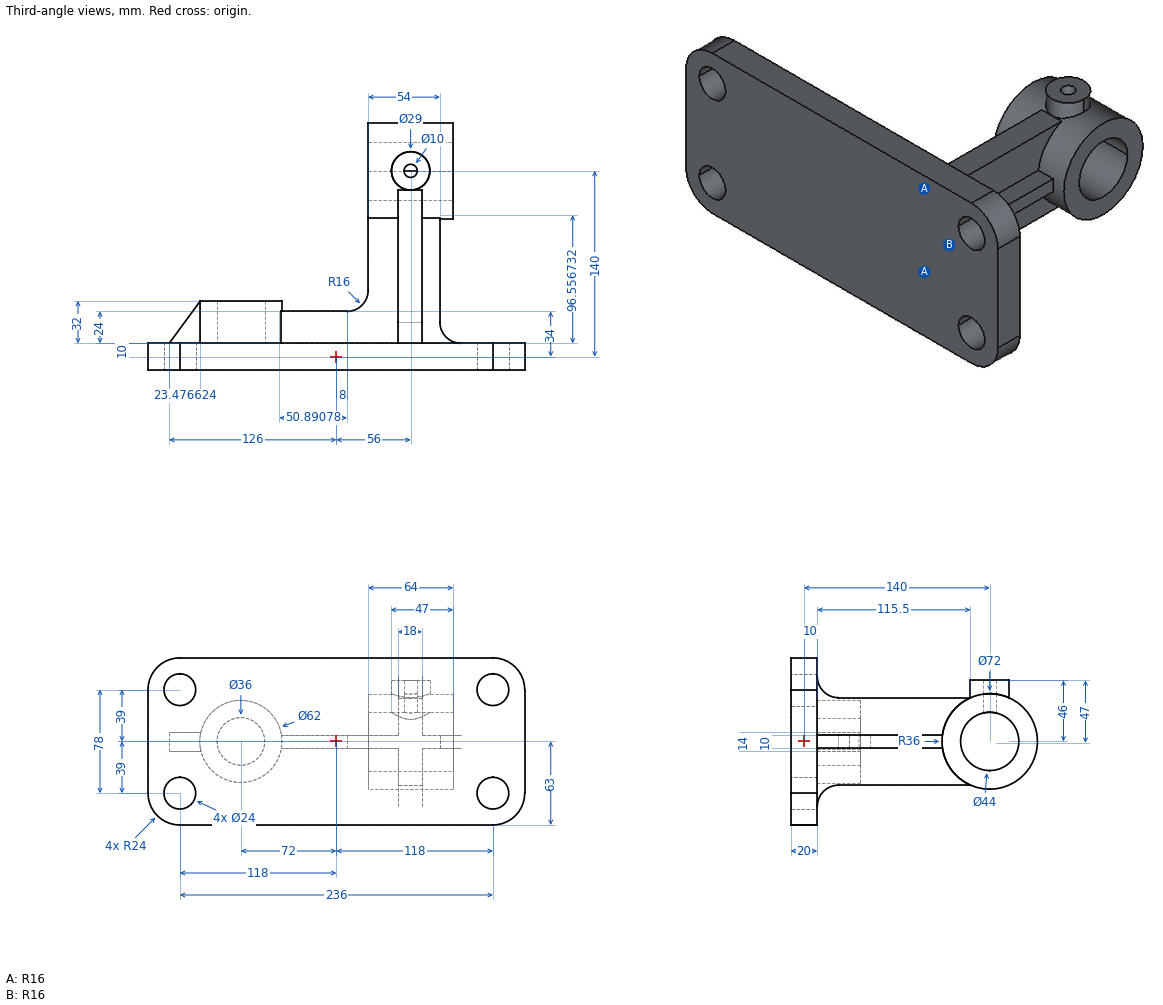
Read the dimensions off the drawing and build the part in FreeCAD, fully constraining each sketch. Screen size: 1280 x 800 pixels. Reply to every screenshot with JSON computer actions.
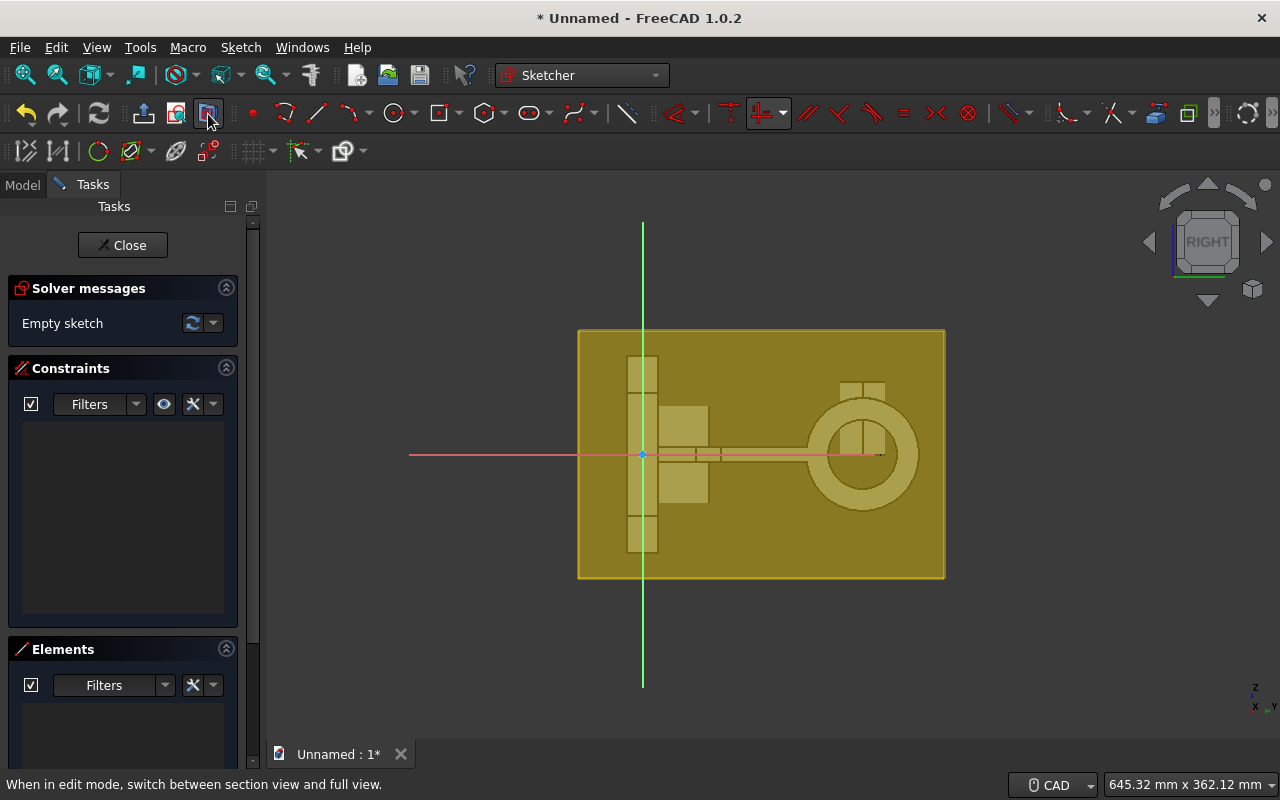
{"action": "scroll", "coordinate": [763, 455], "scroll_direction": "up", "scroll_amount": 5}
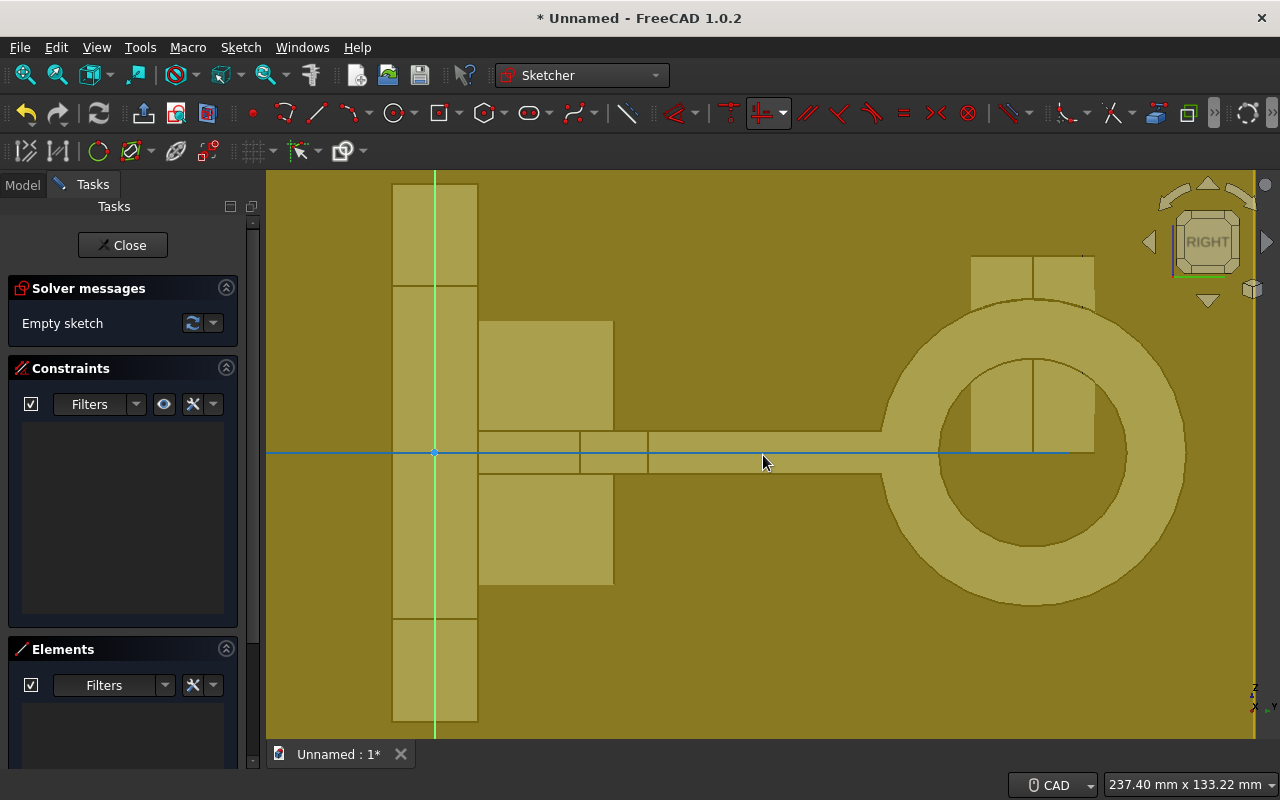
{"action": "left_click", "coordinate": [286, 114]}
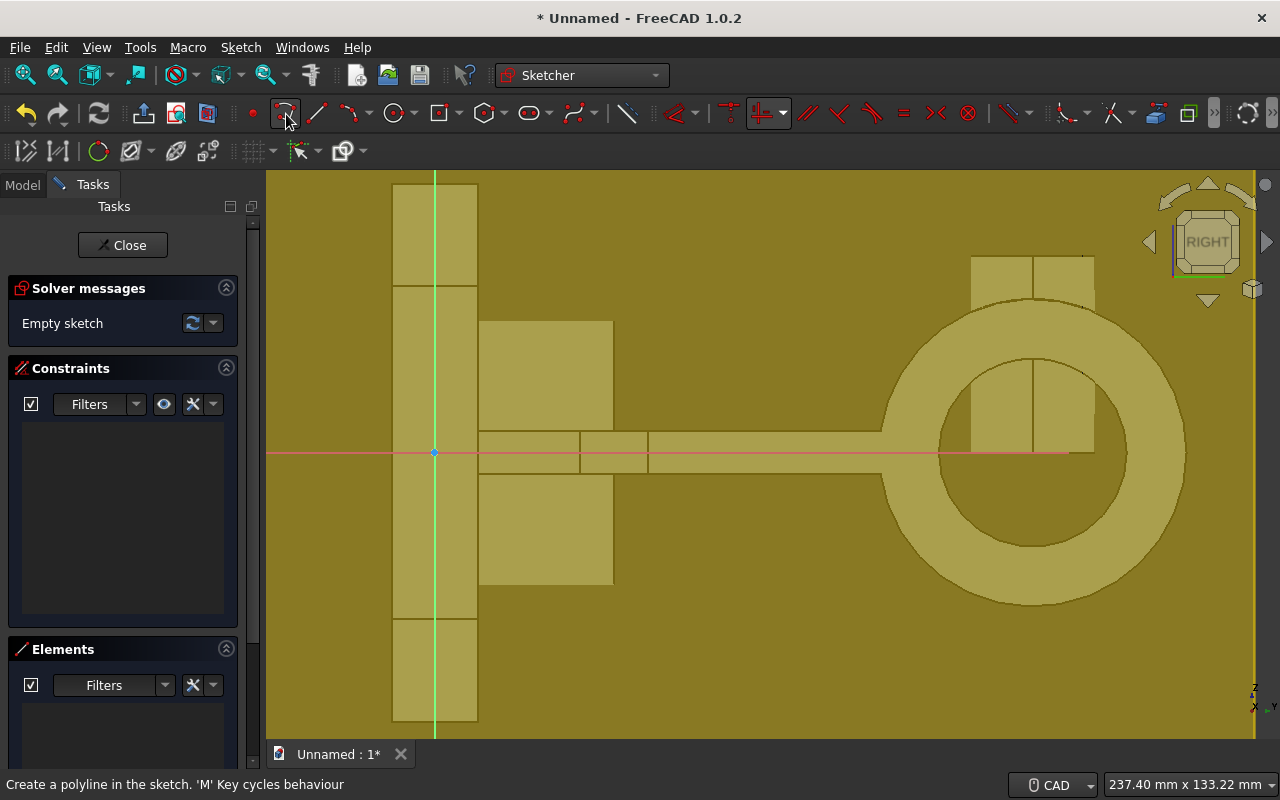
{"action": "left_click", "coordinate": [971, 312]}
{"action": "left_click", "coordinate": [478, 312]}
{"action": "left_click", "coordinate": [478, 594]}
{"action": "left_click", "coordinate": [971, 594]}
{"action": "right_click", "coordinate": [971, 594]}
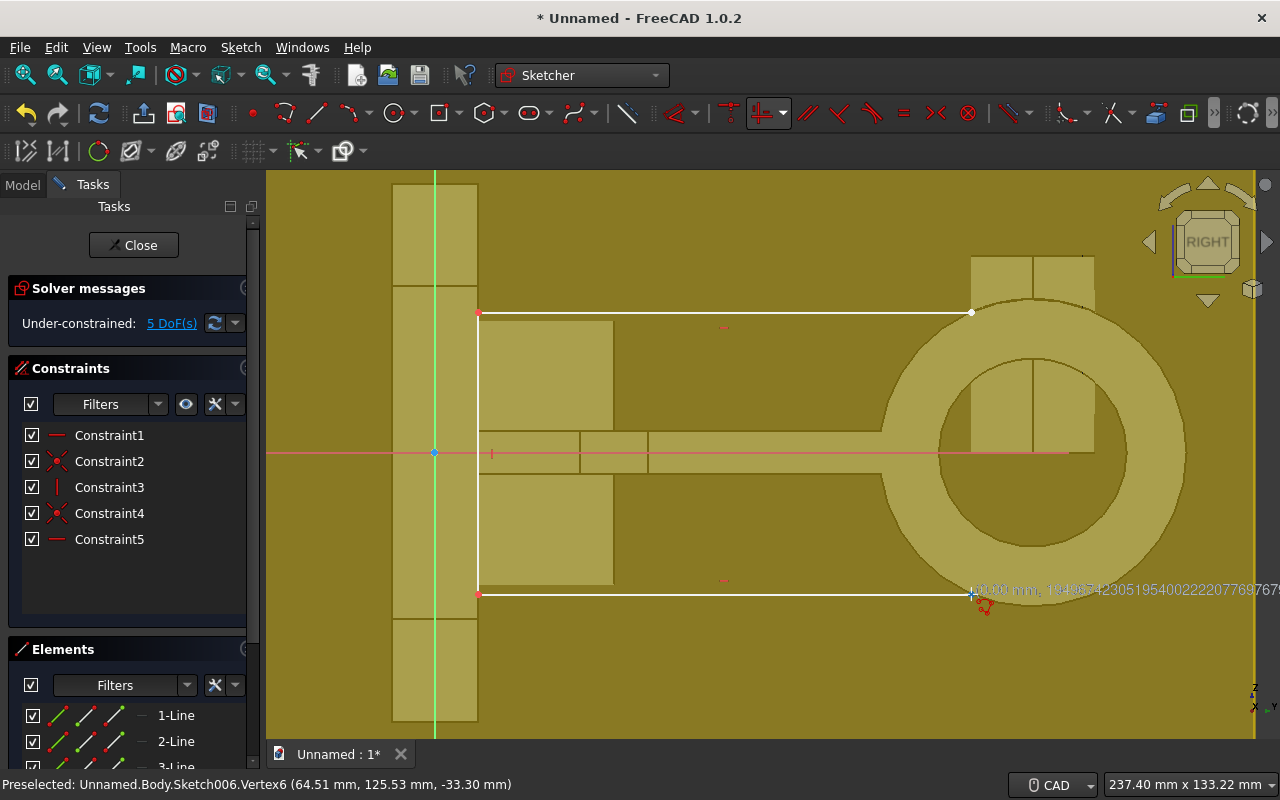
{"action": "left_click", "coordinate": [350, 114]}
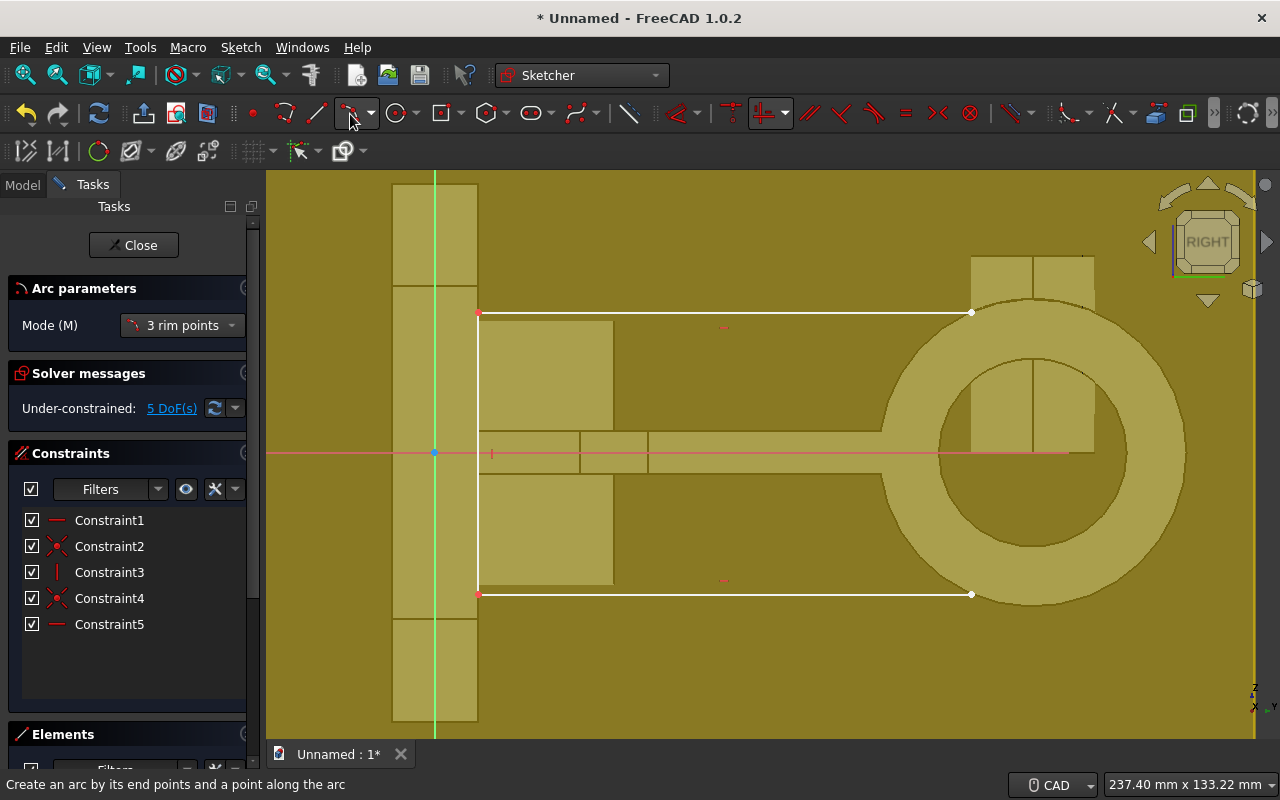
{"action": "left_click", "coordinate": [971, 595]}
{"action": "left_click", "coordinate": [971, 313]}
{"action": "left_click", "coordinate": [883, 418]}
{"action": "key", "text": "Escape"}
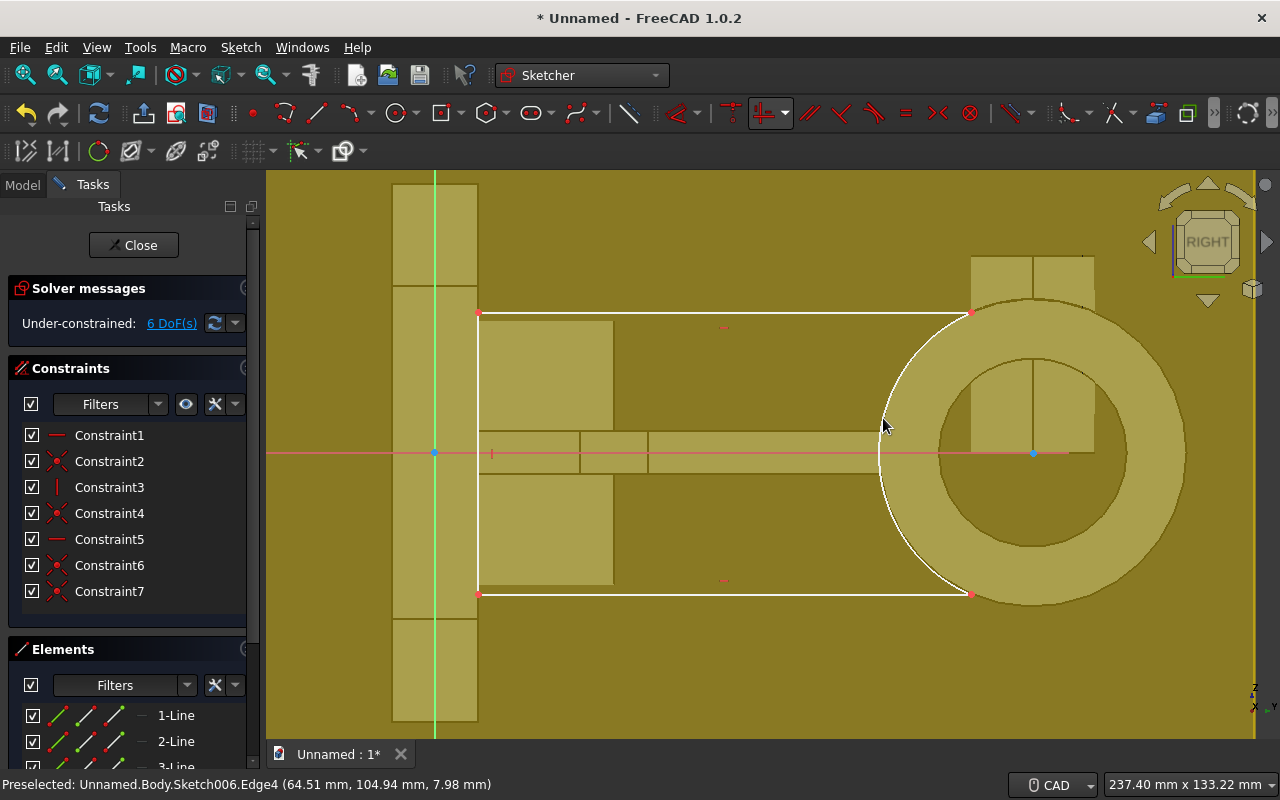
{"action": "left_click", "coordinate": [1033, 454]}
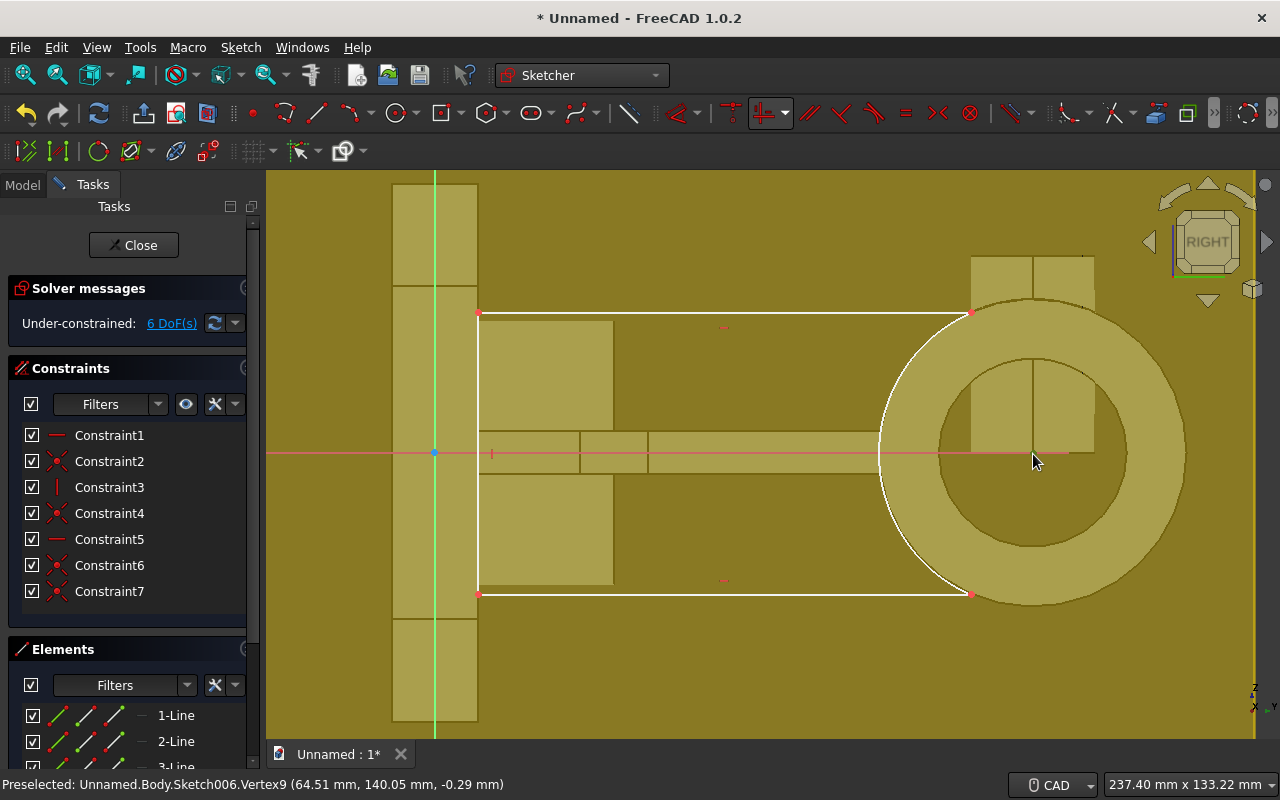
{"action": "left_click", "coordinate": [353, 453]}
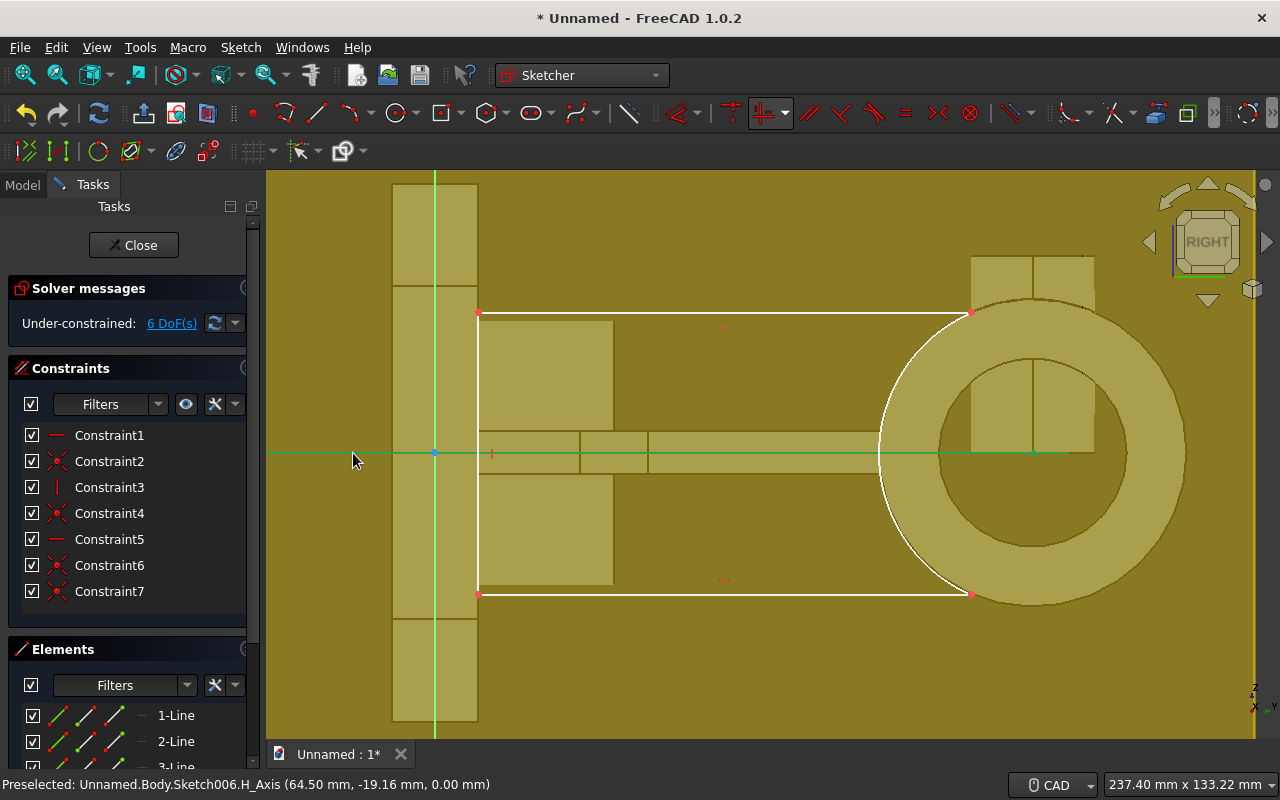
{"action": "left_click", "coordinate": [732, 114]}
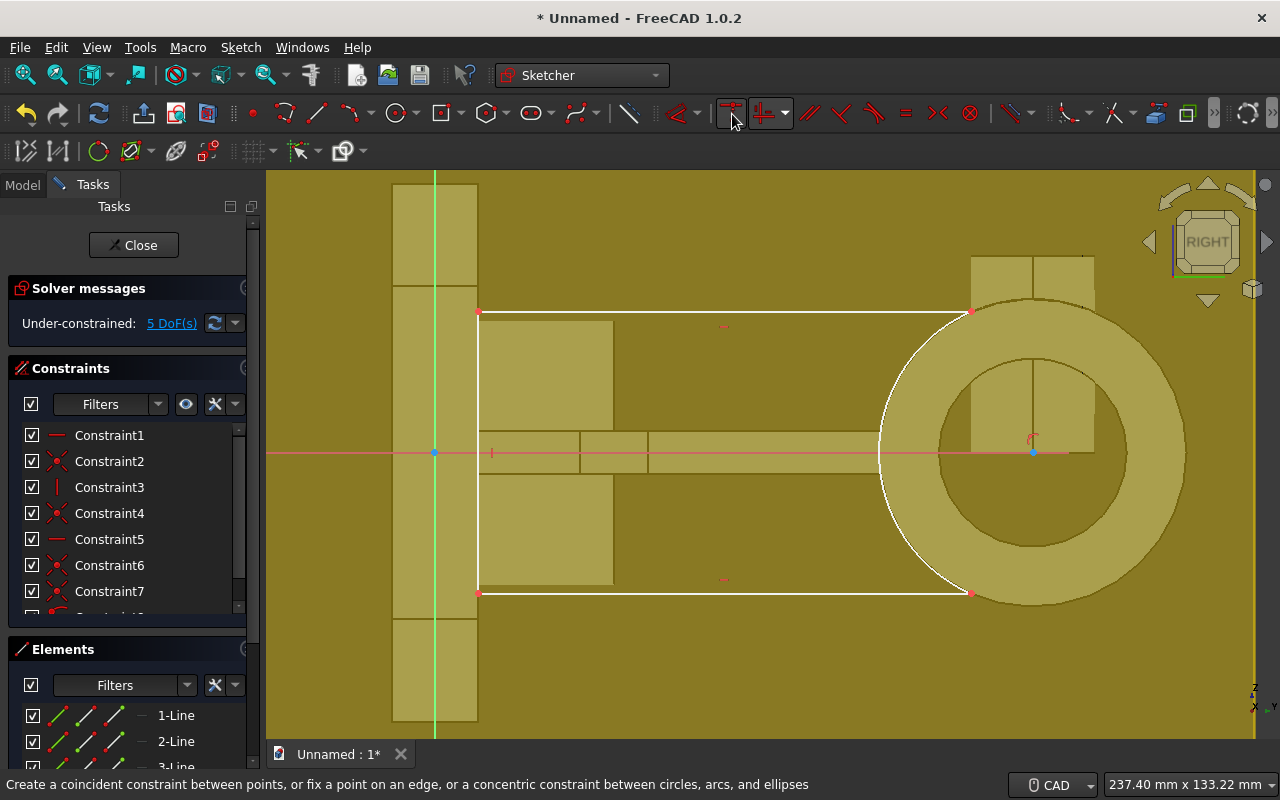
{"action": "left_click", "coordinate": [676, 114]}